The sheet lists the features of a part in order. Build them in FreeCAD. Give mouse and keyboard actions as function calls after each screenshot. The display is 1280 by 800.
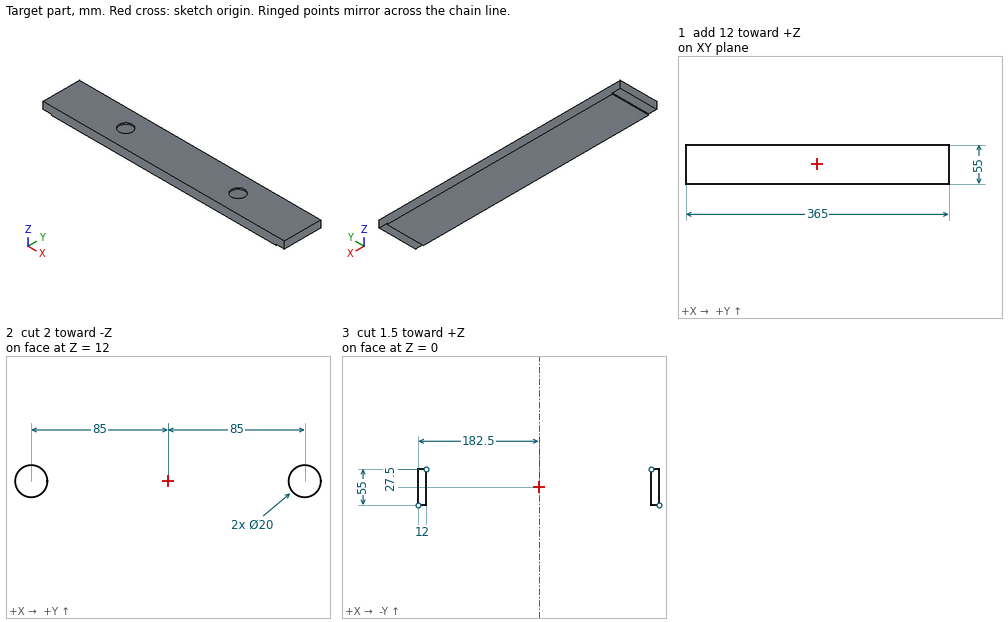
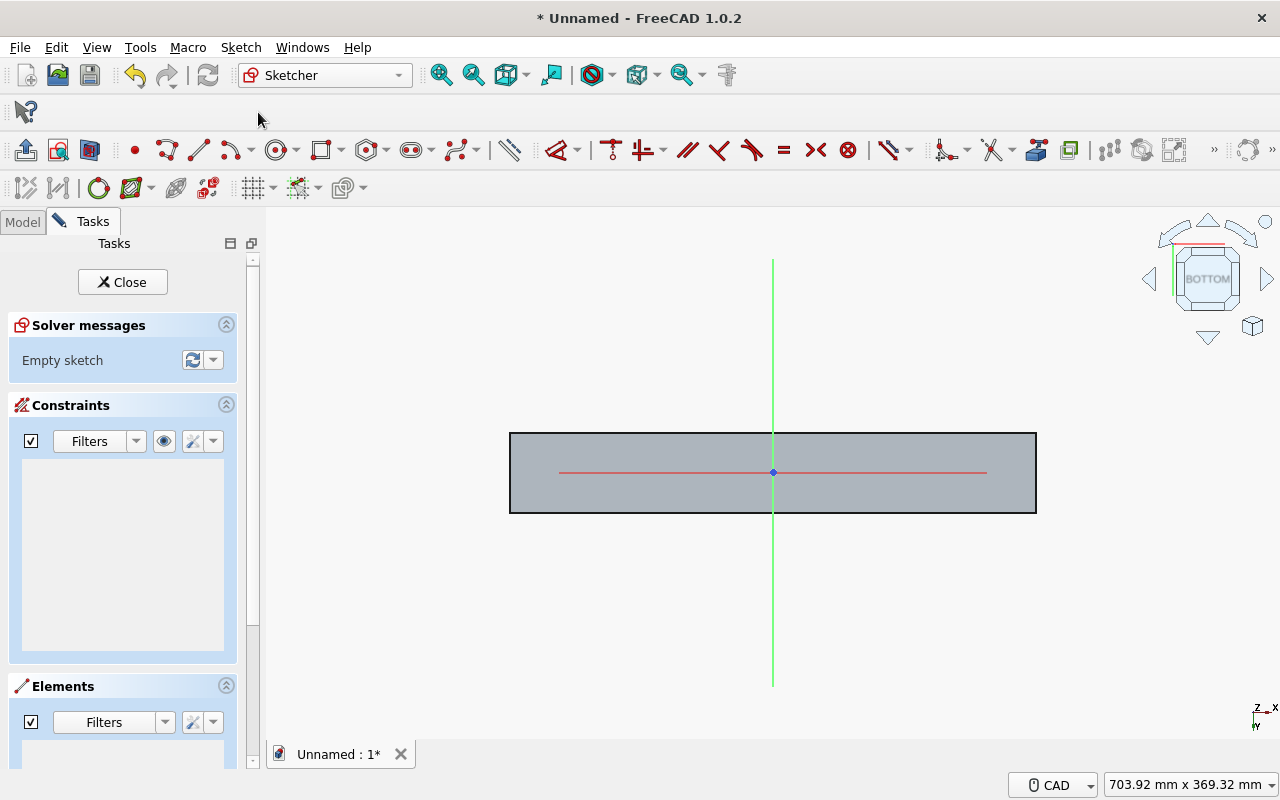
key(g)
key(r)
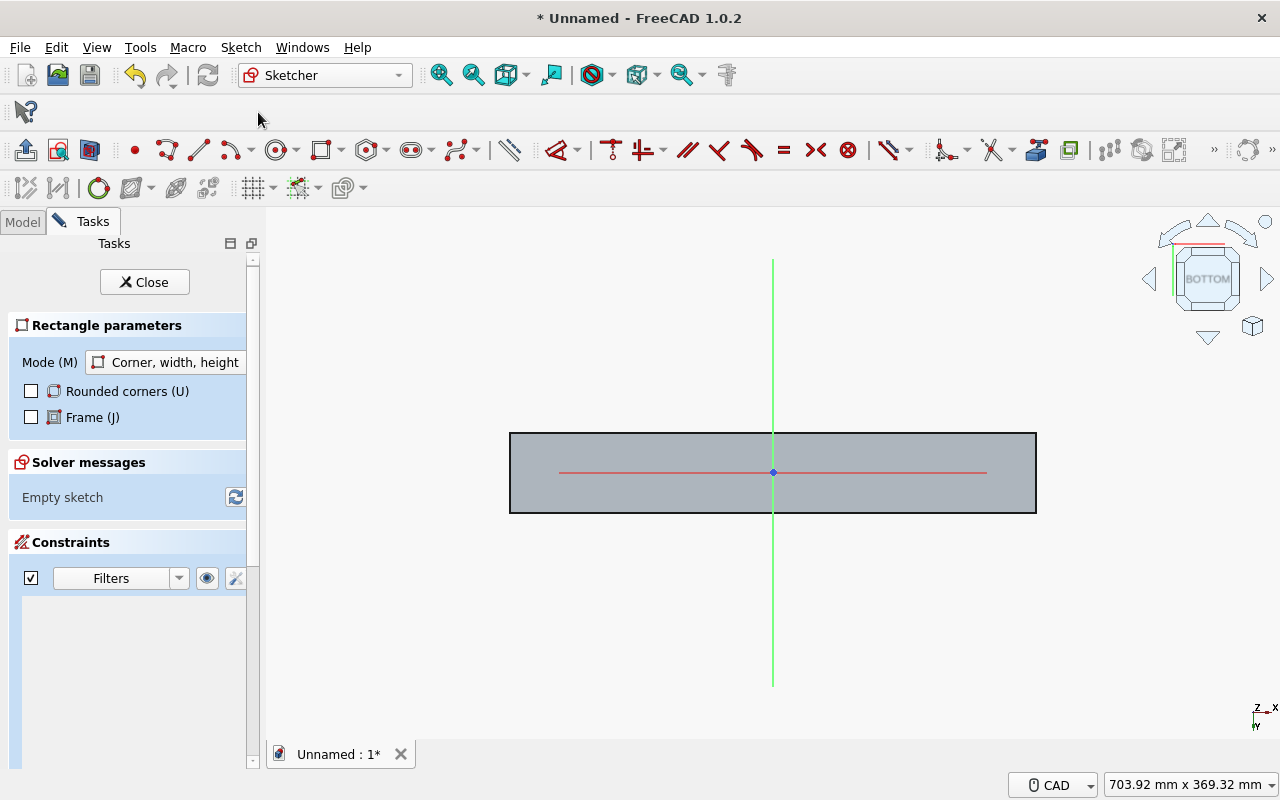
click(510, 433)
click(527, 513)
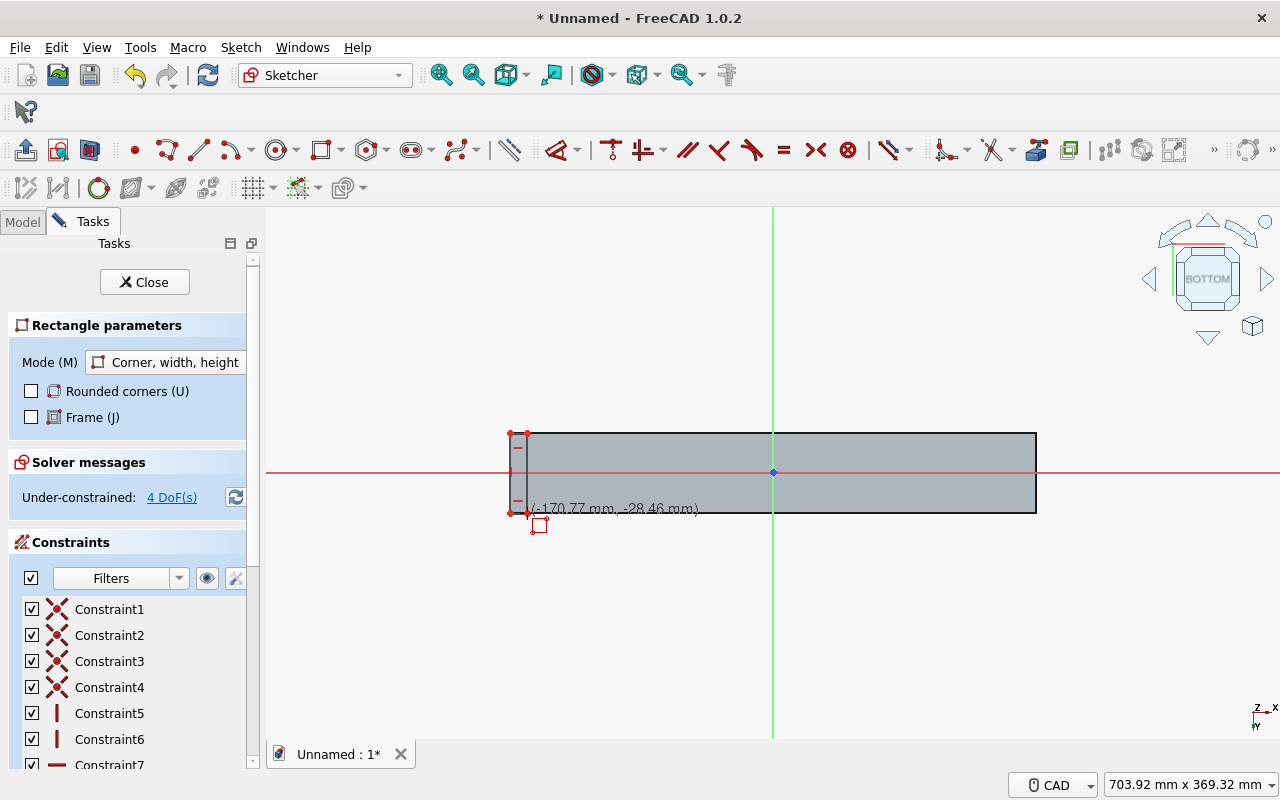
click(1019, 433)
click(1036, 513)
key(Escape)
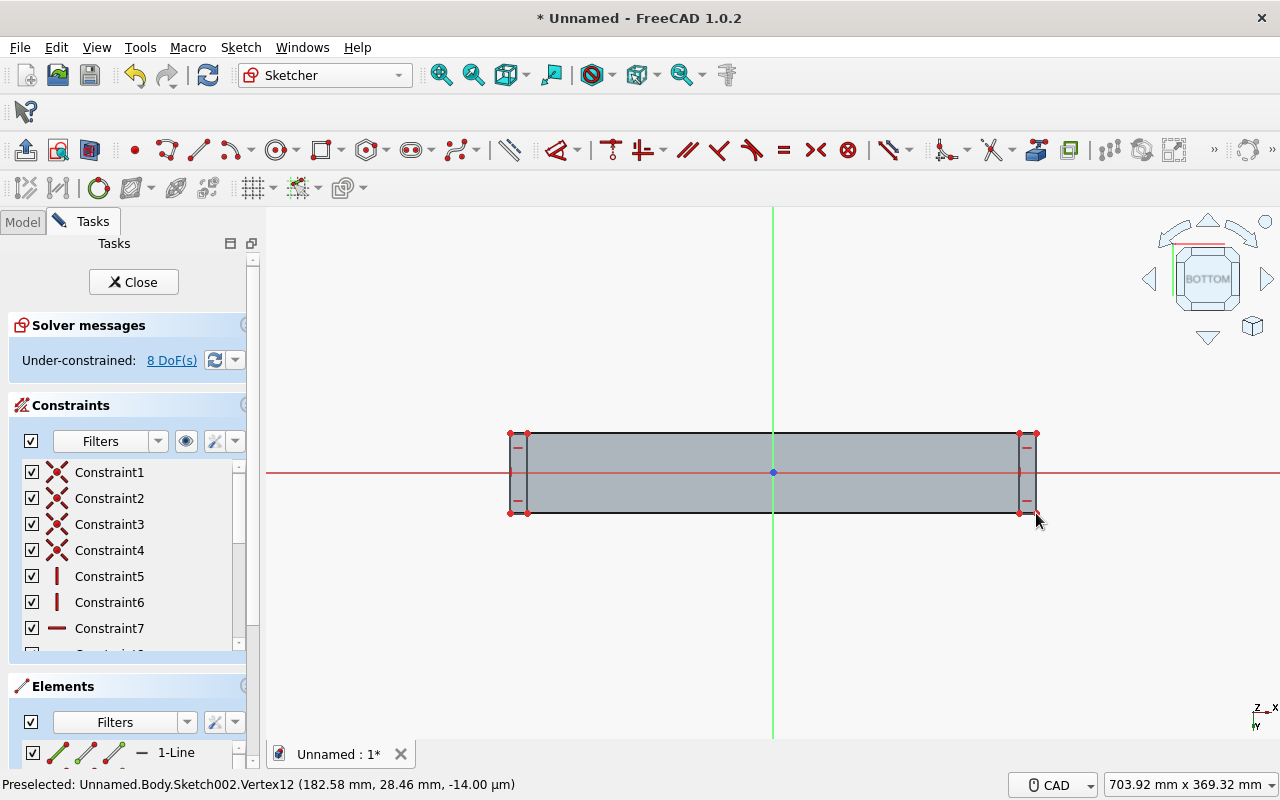
click(527, 434)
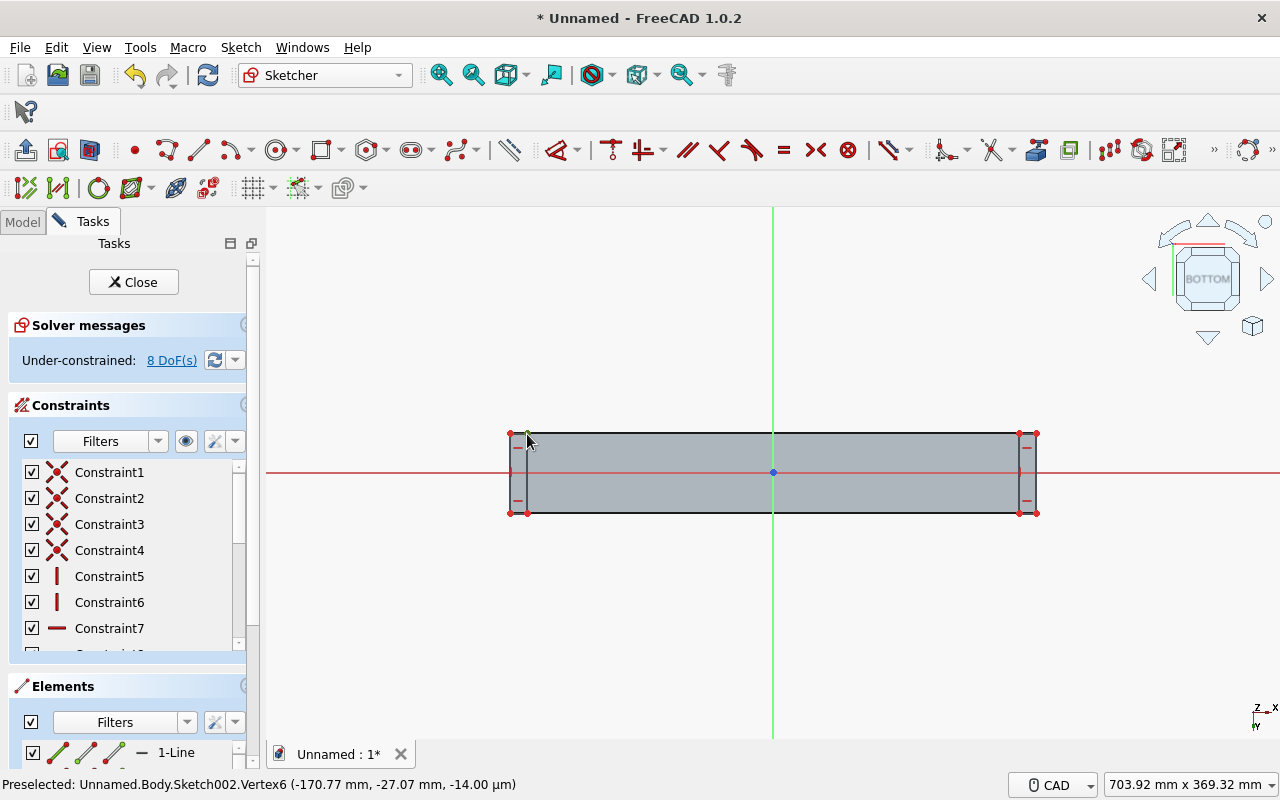
click(1019, 434)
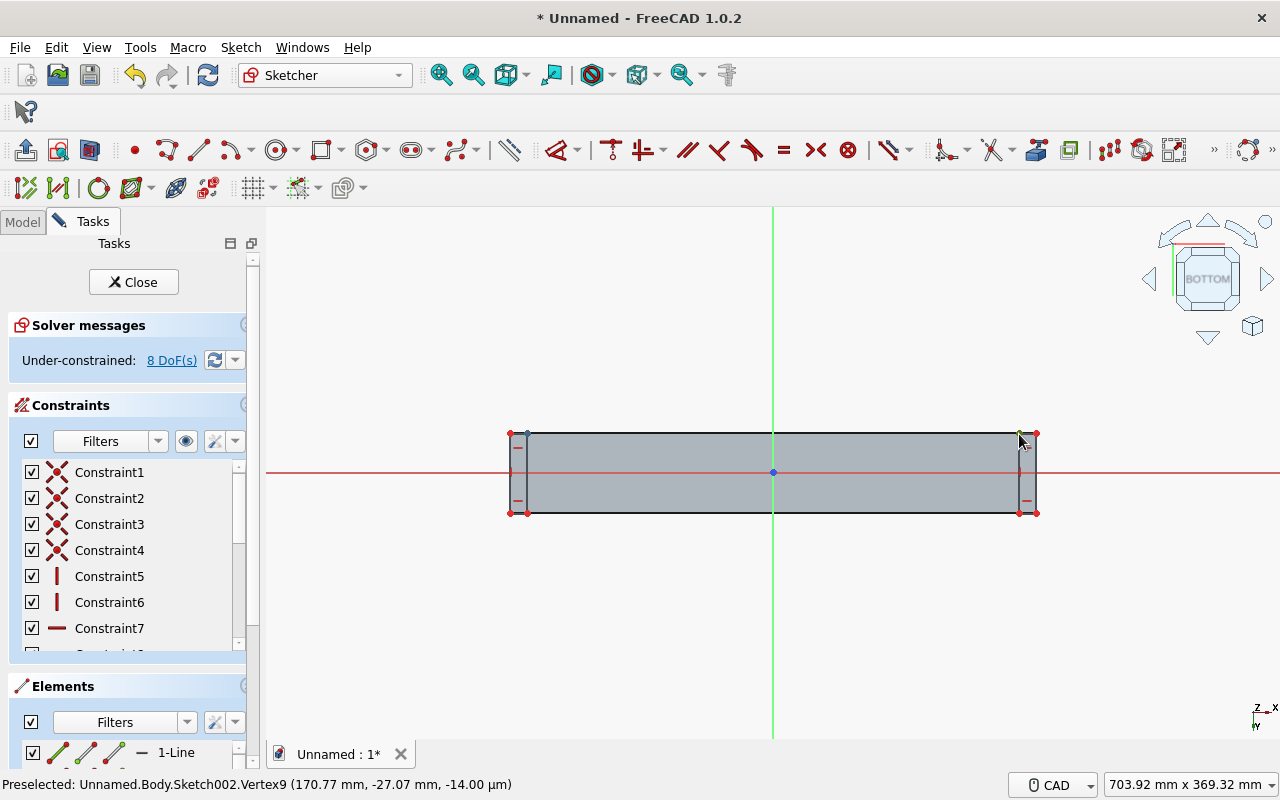
click(773, 677)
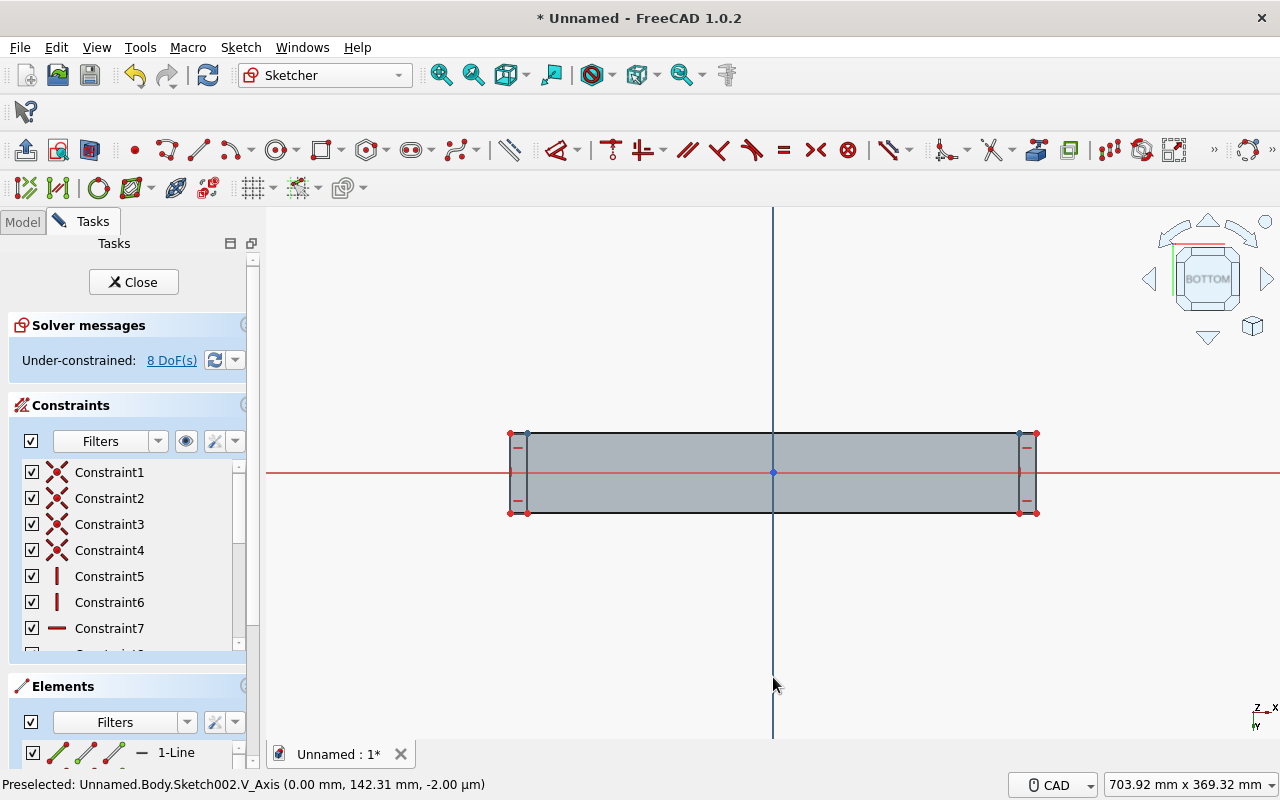
click(816, 150)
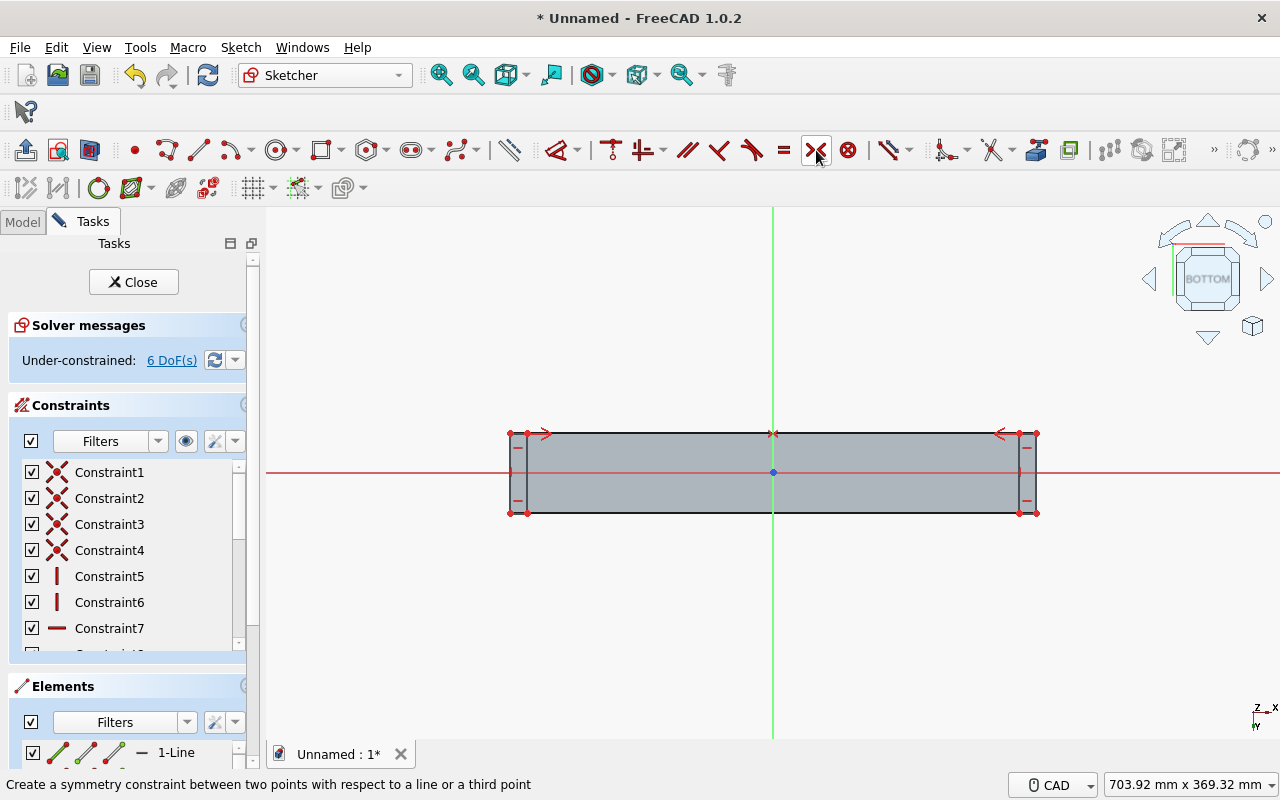
click(510, 514)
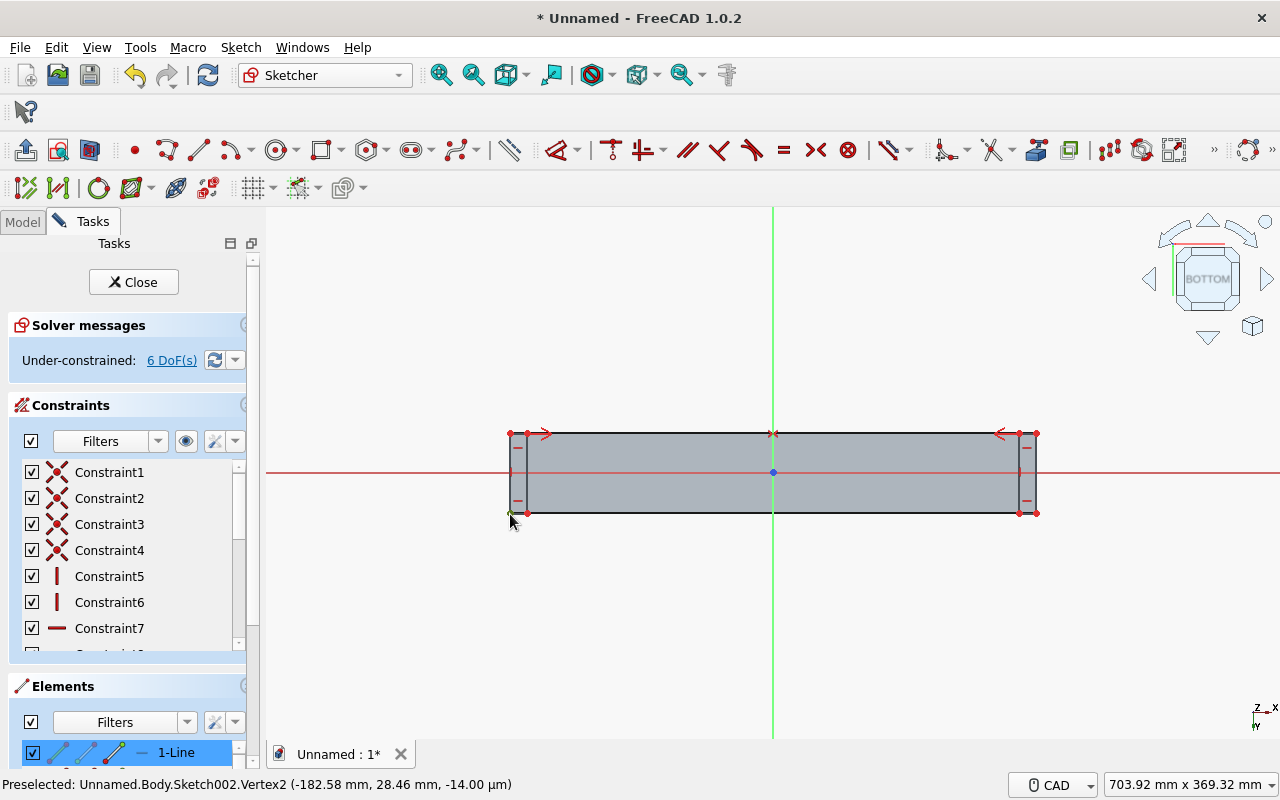
click(1036, 514)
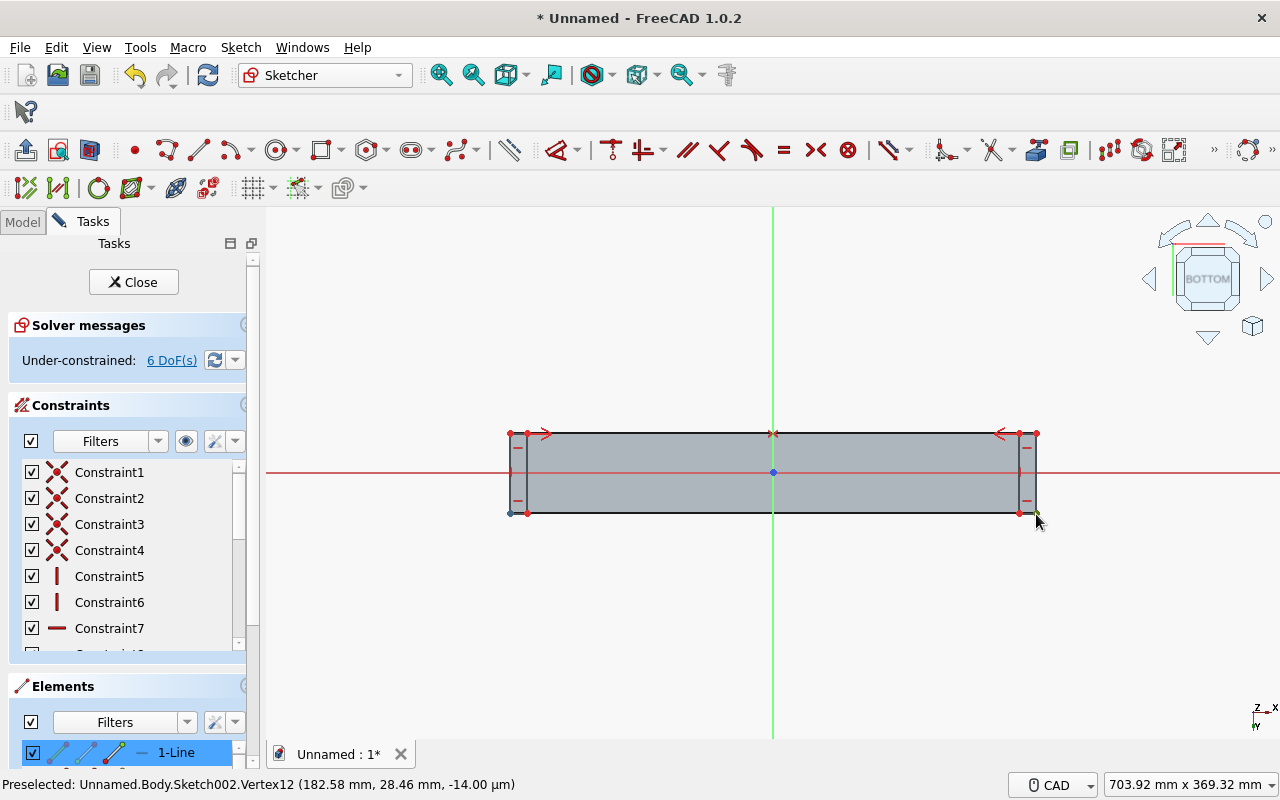
click(773, 677)